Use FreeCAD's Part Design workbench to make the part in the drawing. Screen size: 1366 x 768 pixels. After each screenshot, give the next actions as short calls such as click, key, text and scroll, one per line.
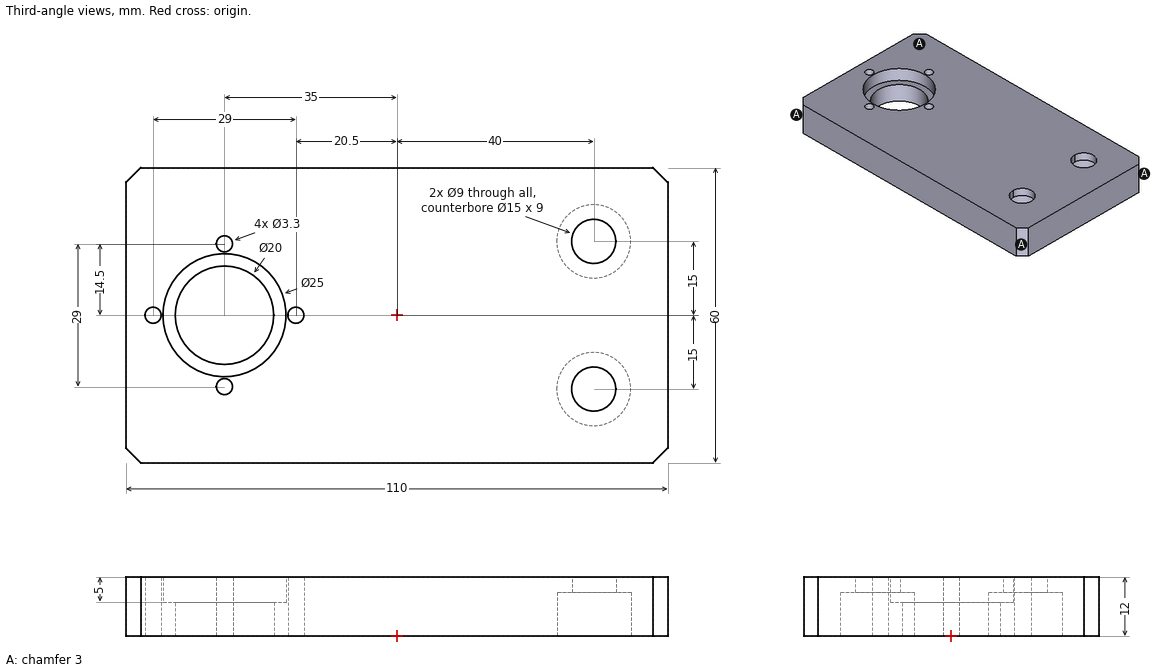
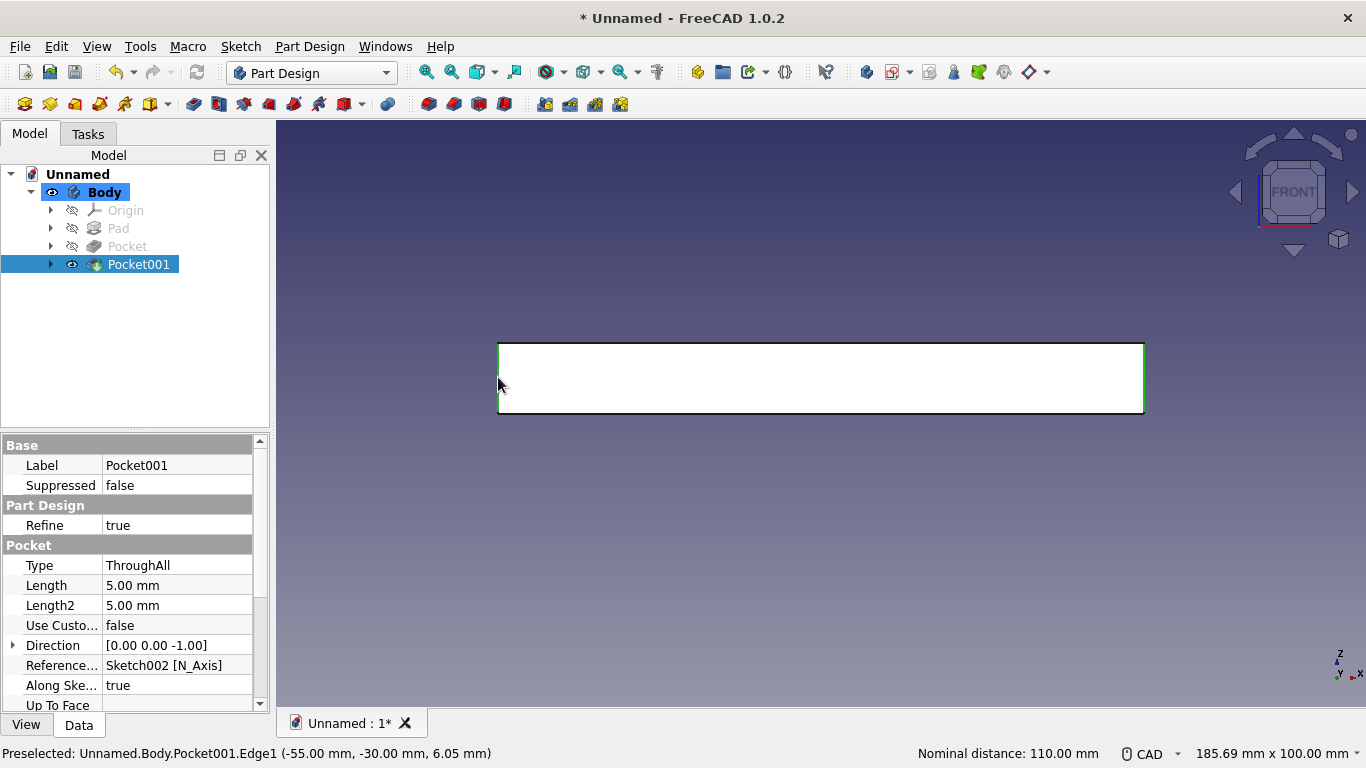
key(3)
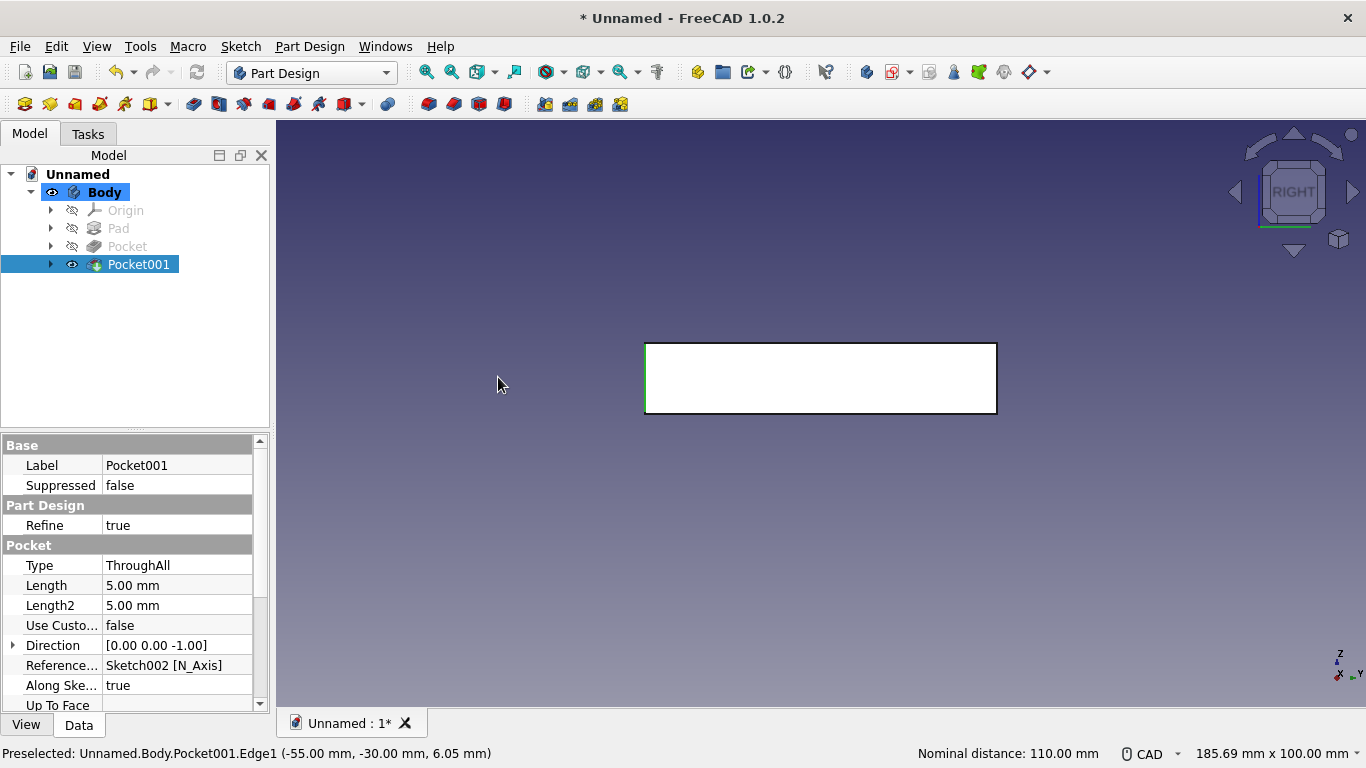
key(v)
key(f)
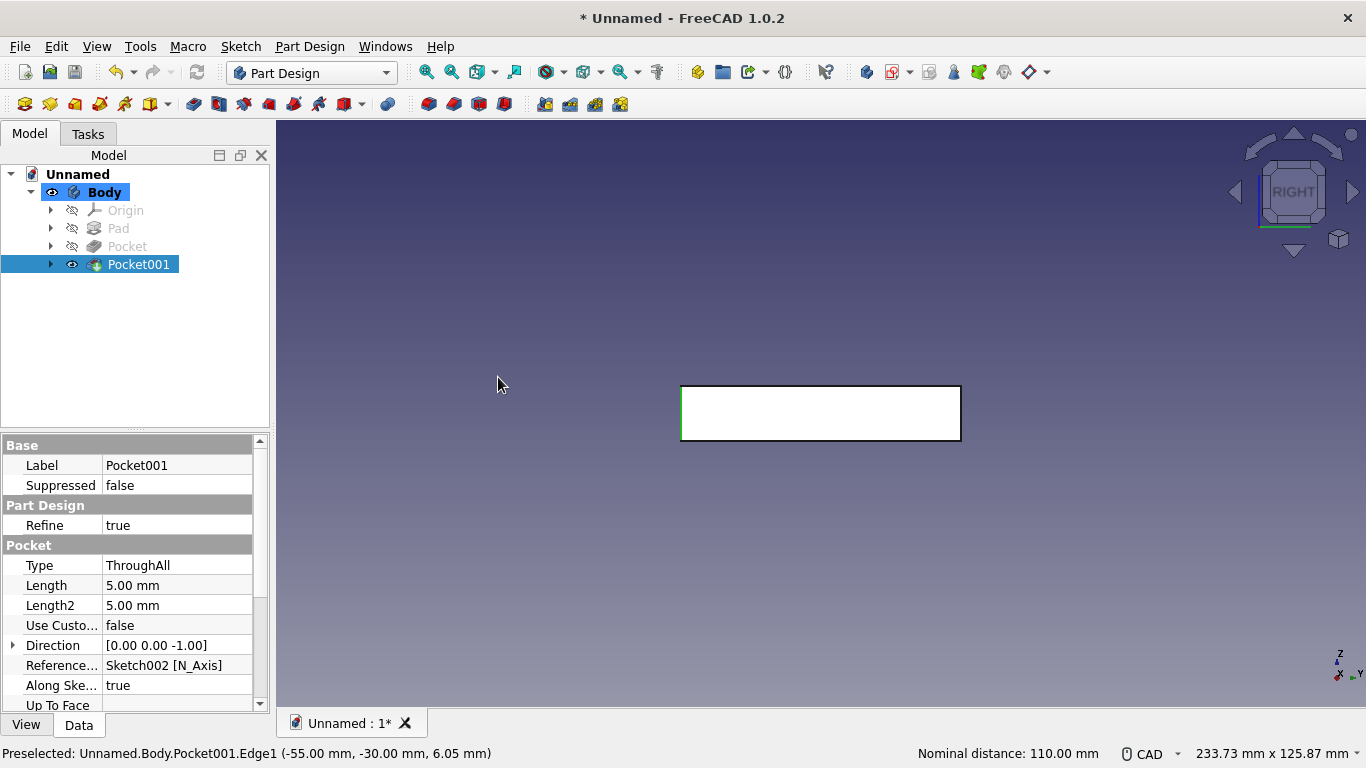
click(961, 412, ctrl)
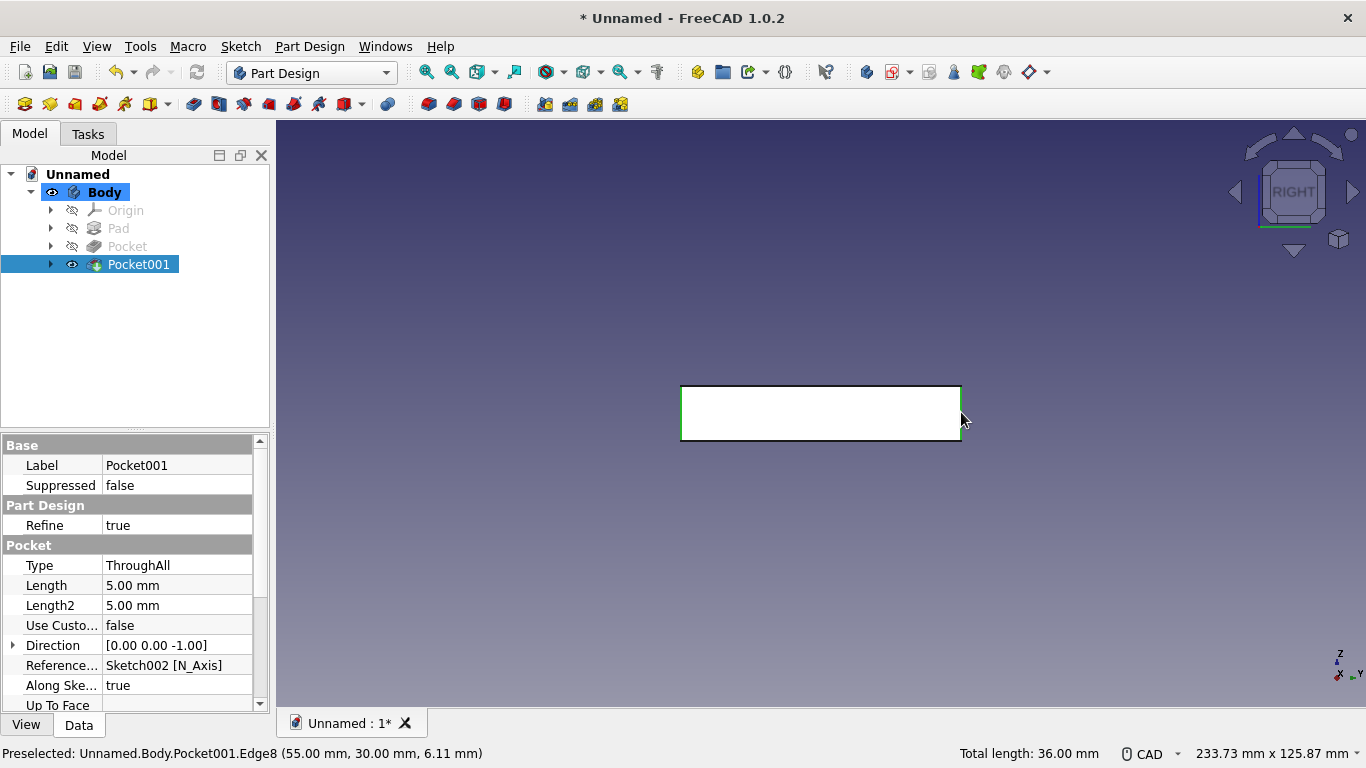
key(5)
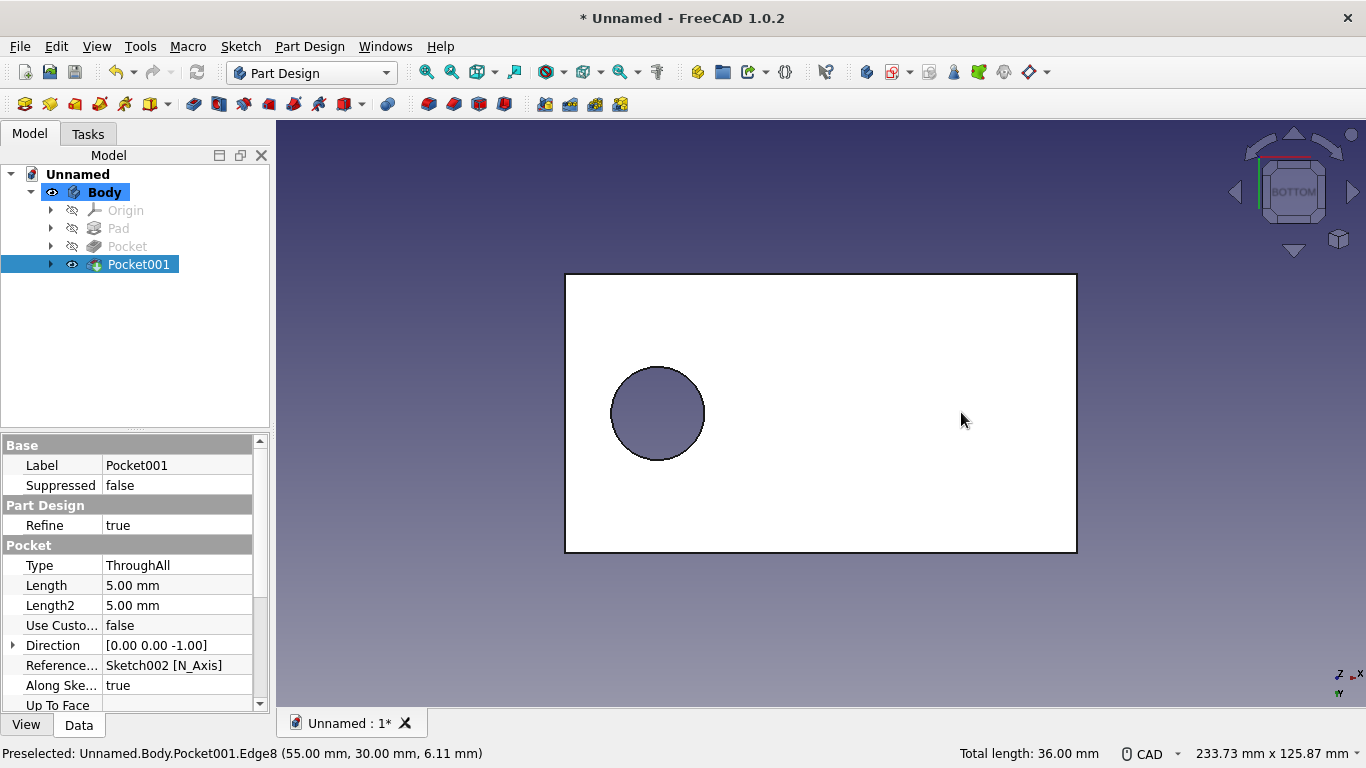
key(4)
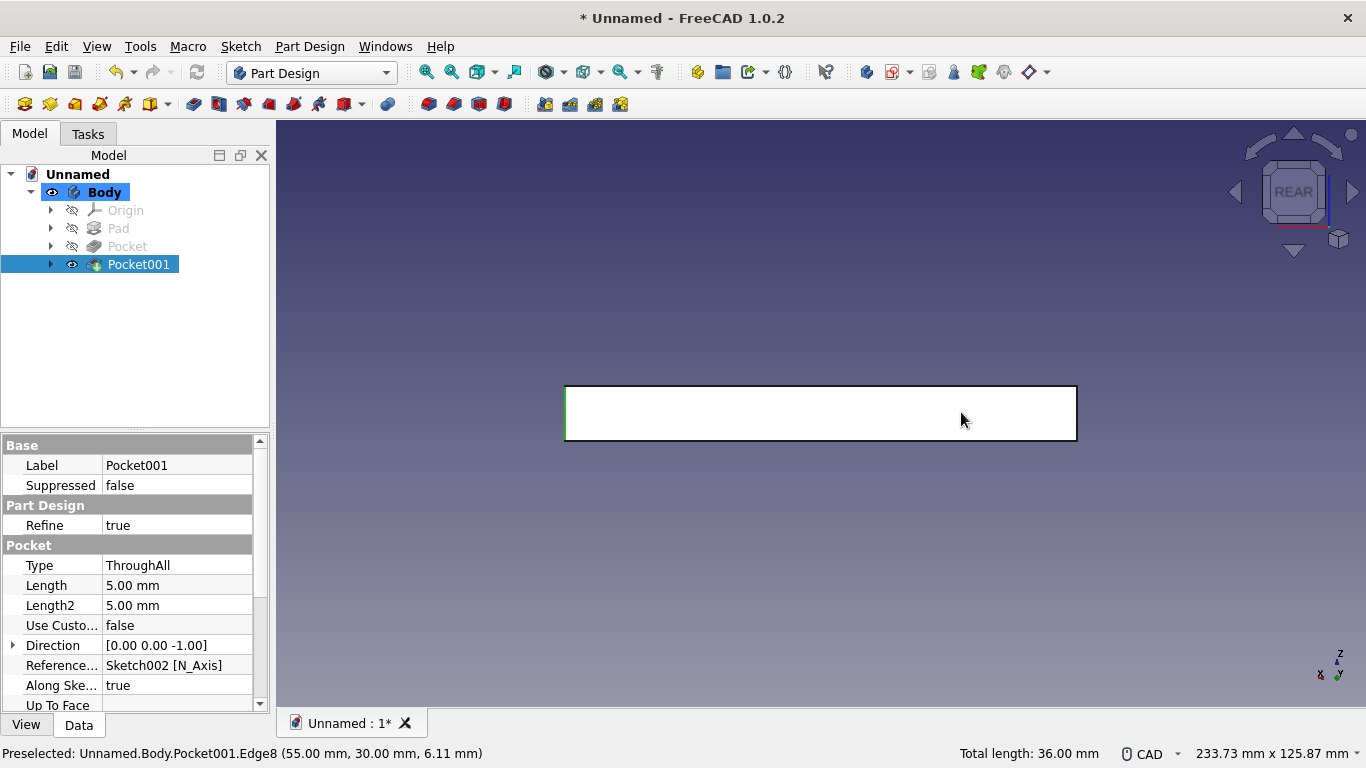
click(1077, 413, ctrl)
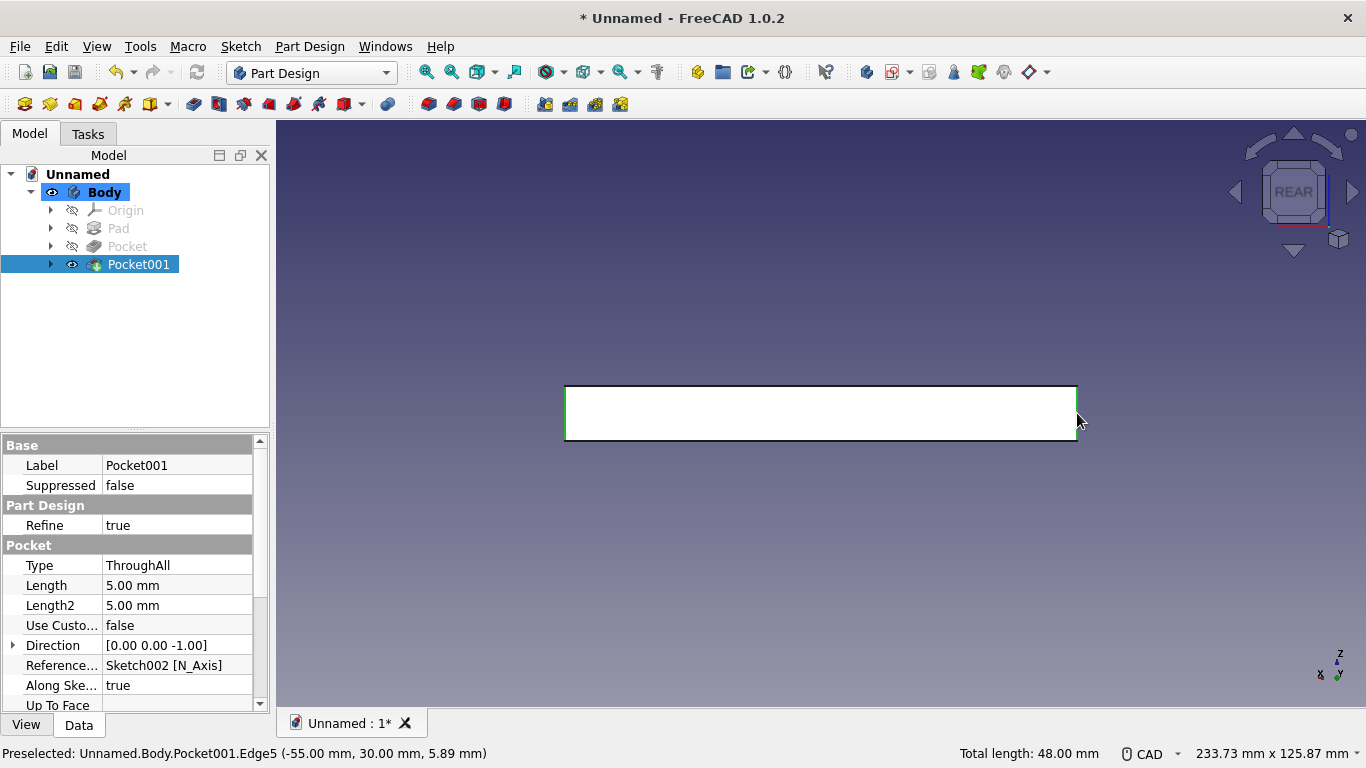
click(454, 104)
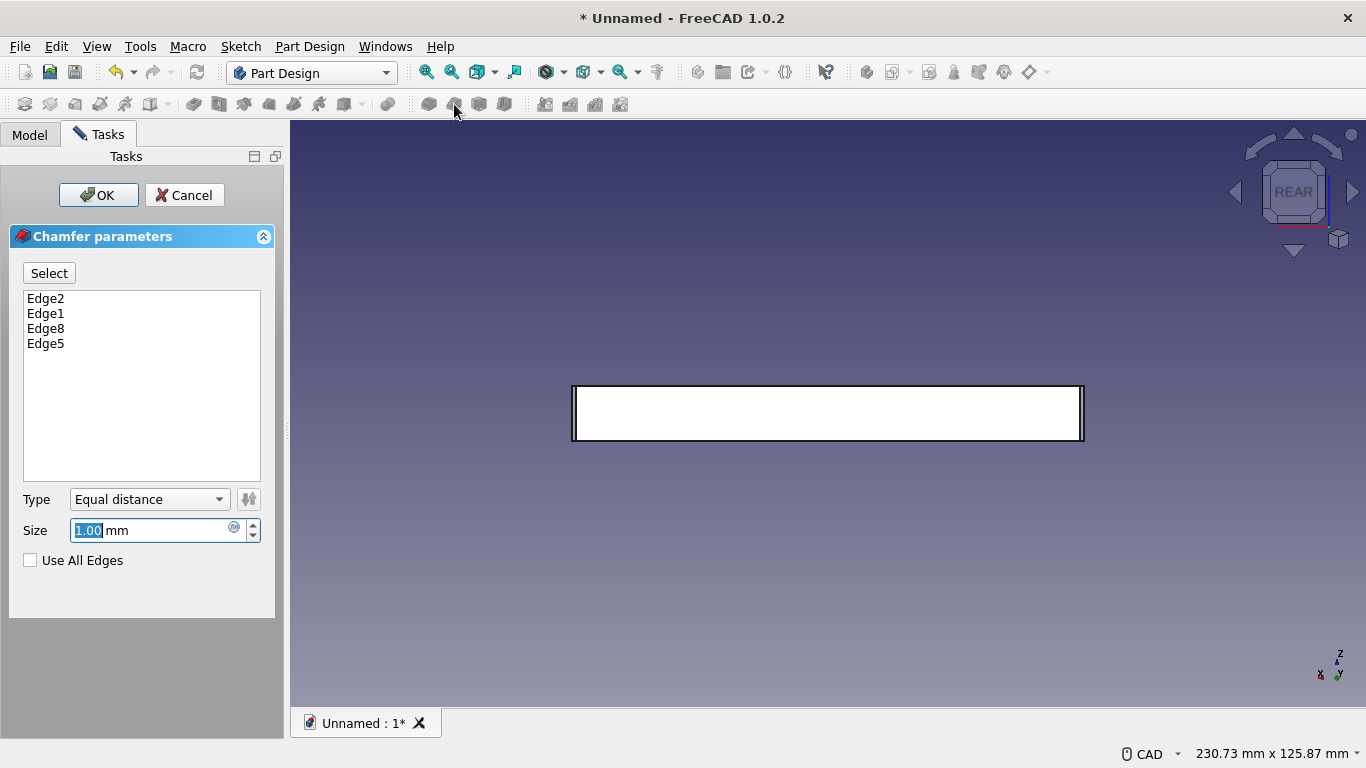
text(3)
key(Tab)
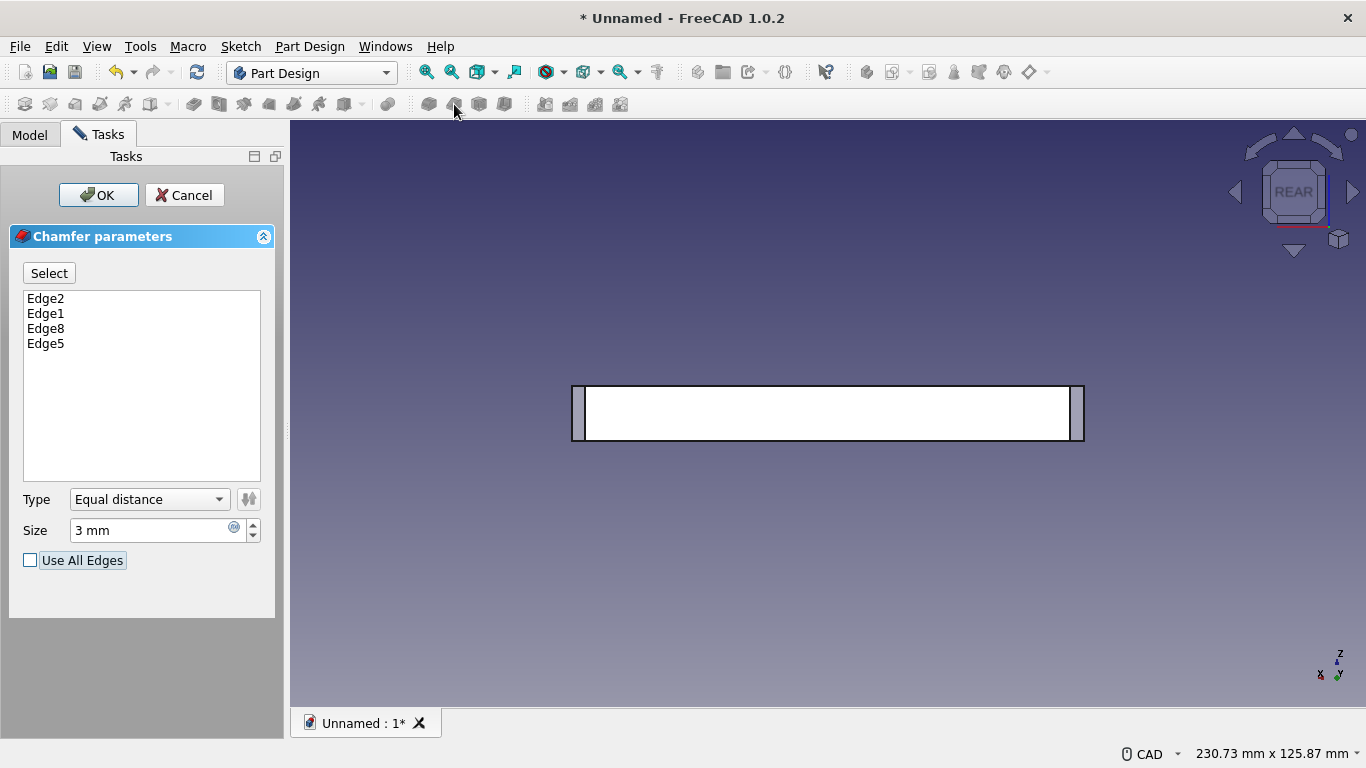
click(99, 195)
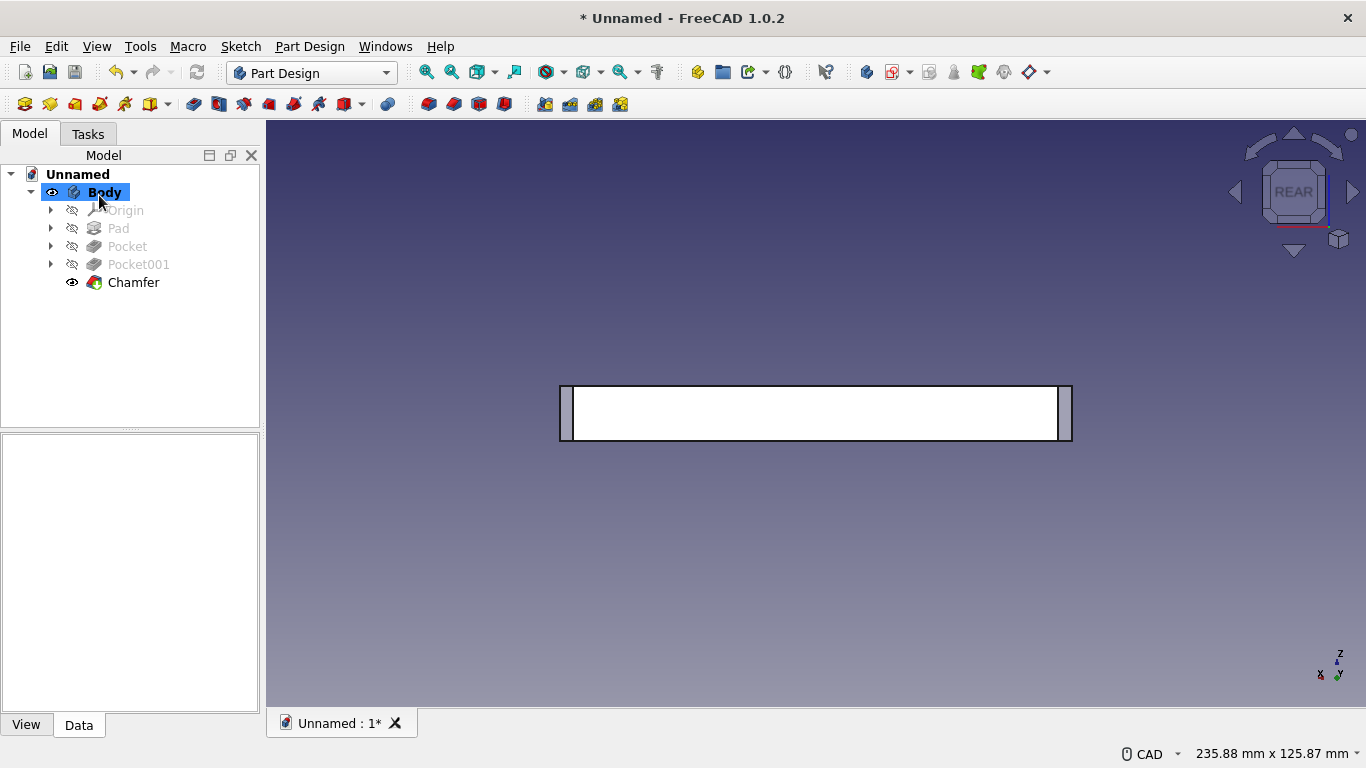
key(0)